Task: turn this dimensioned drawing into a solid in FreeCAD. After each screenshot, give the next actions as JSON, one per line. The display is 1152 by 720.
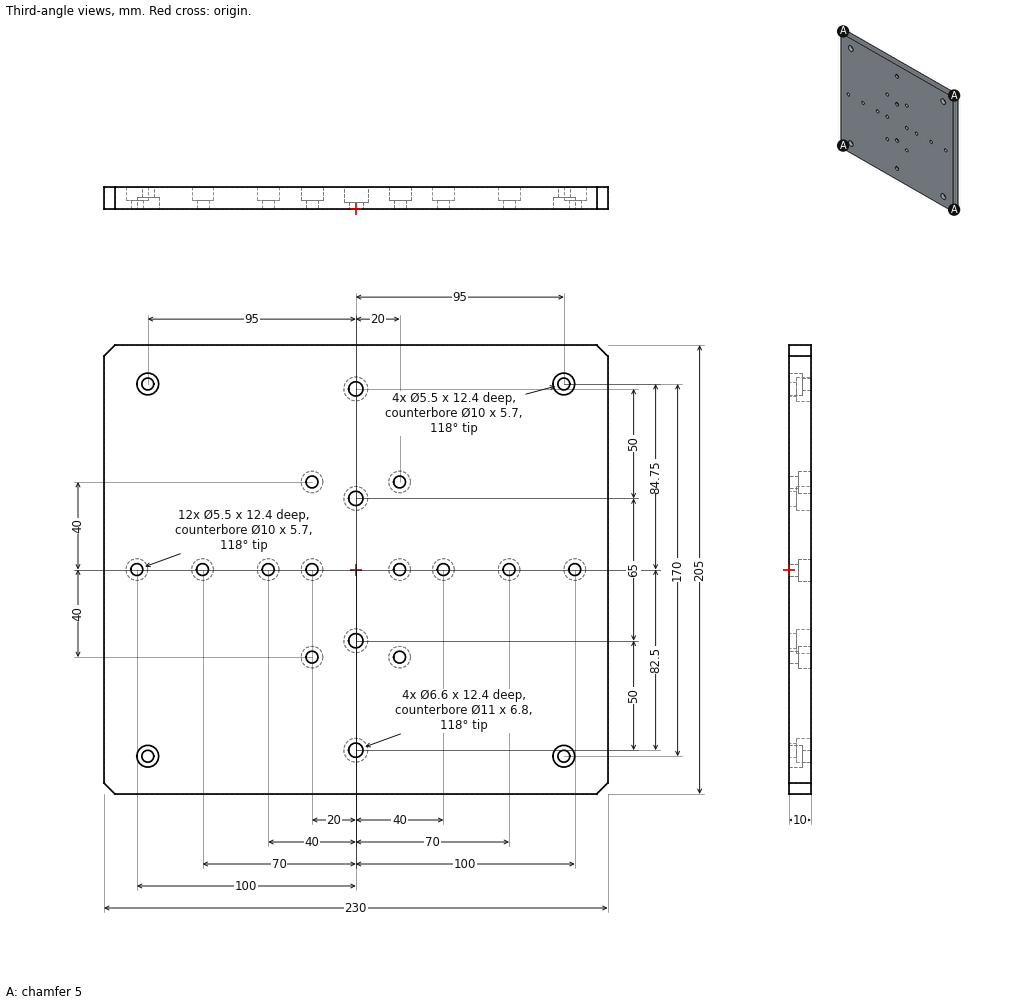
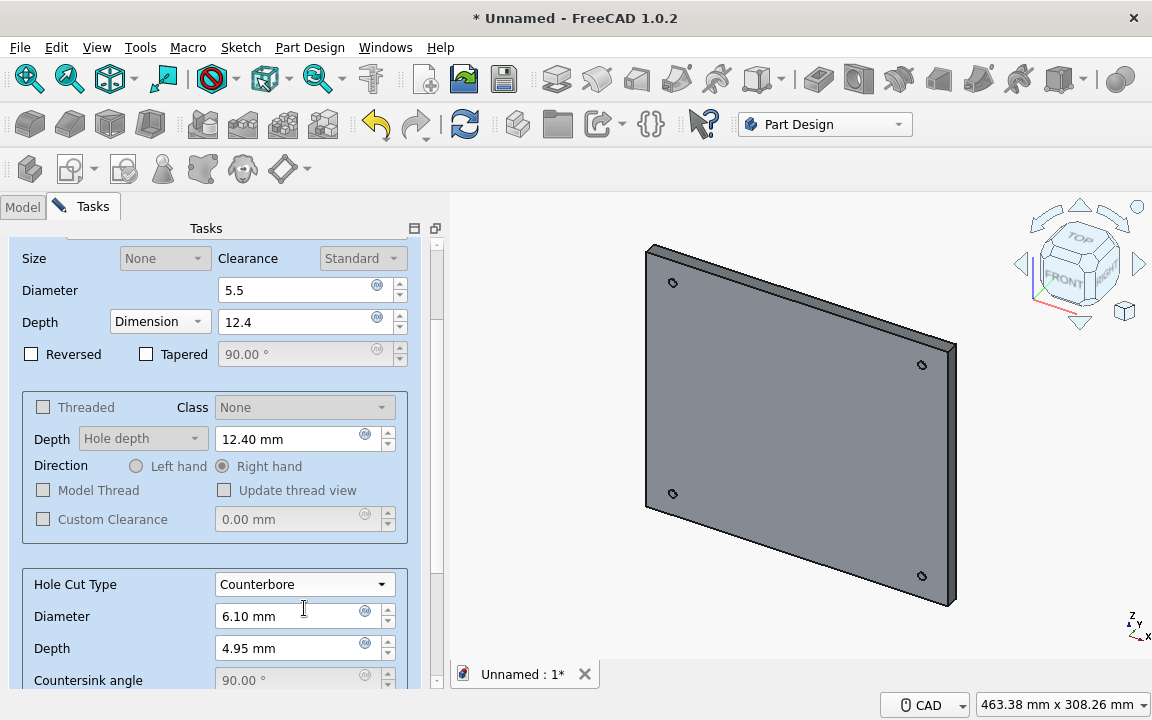
{"action": "triple_click", "coordinate": [298, 616]}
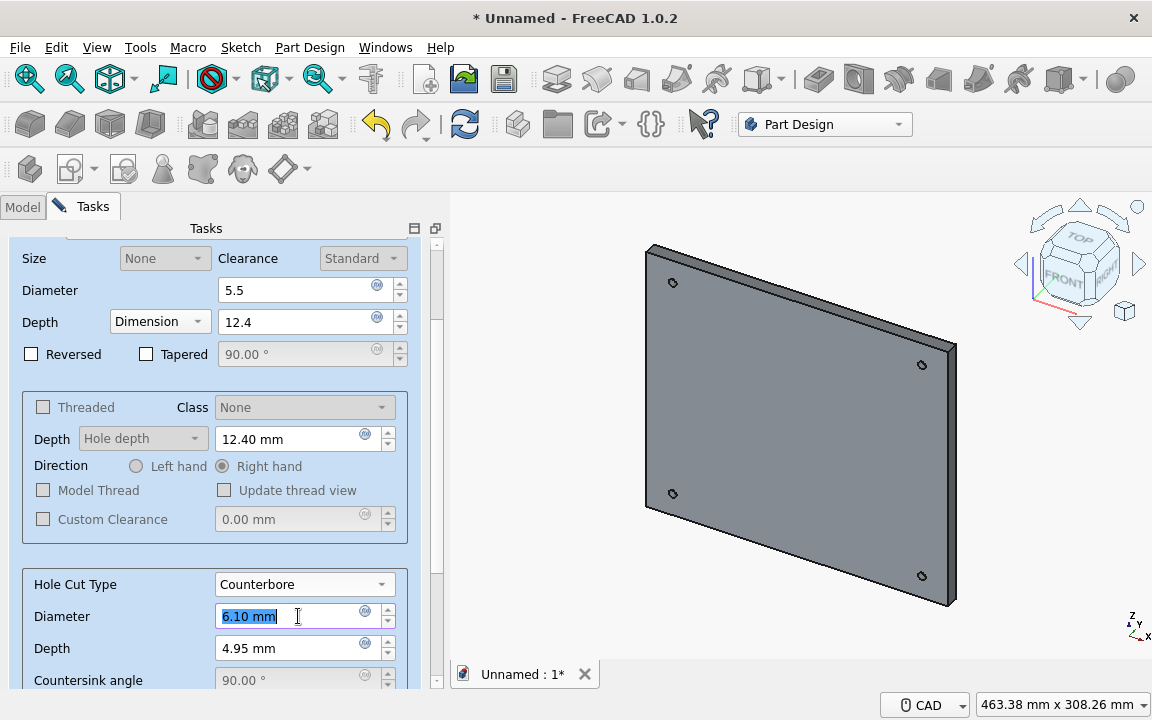
{"action": "type", "text": "10"}
{"action": "key", "text": "Tab"}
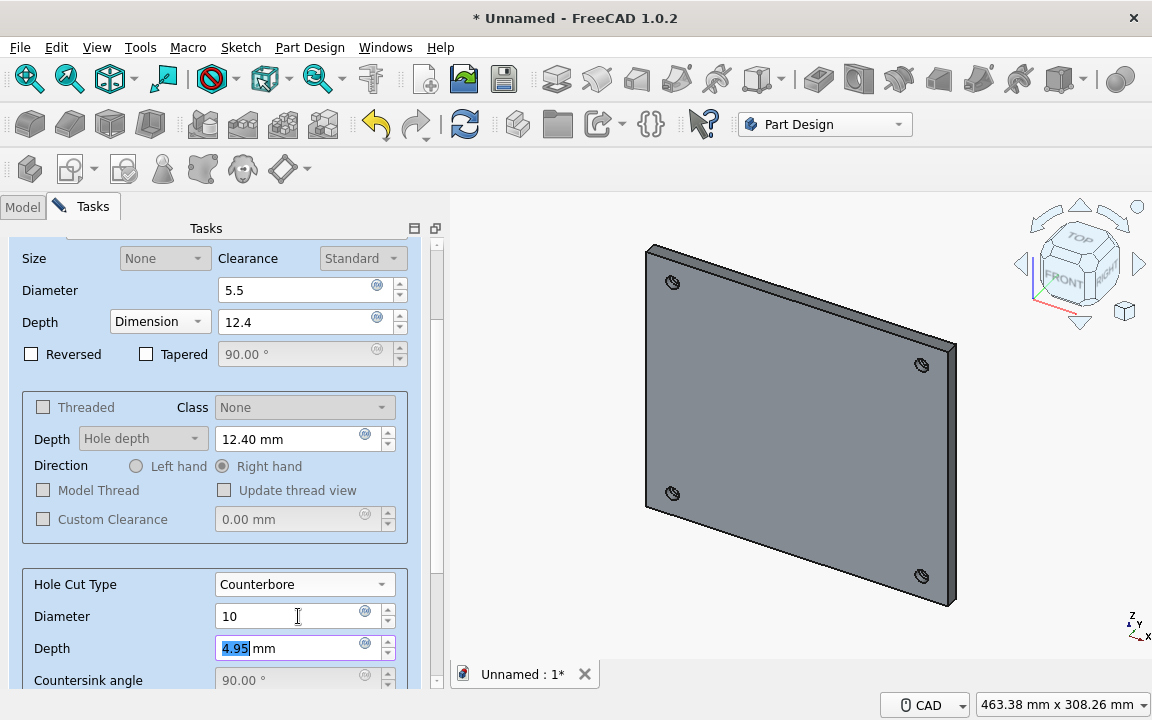
{"action": "type", "text": "5.7"}
{"action": "key", "text": "Tab"}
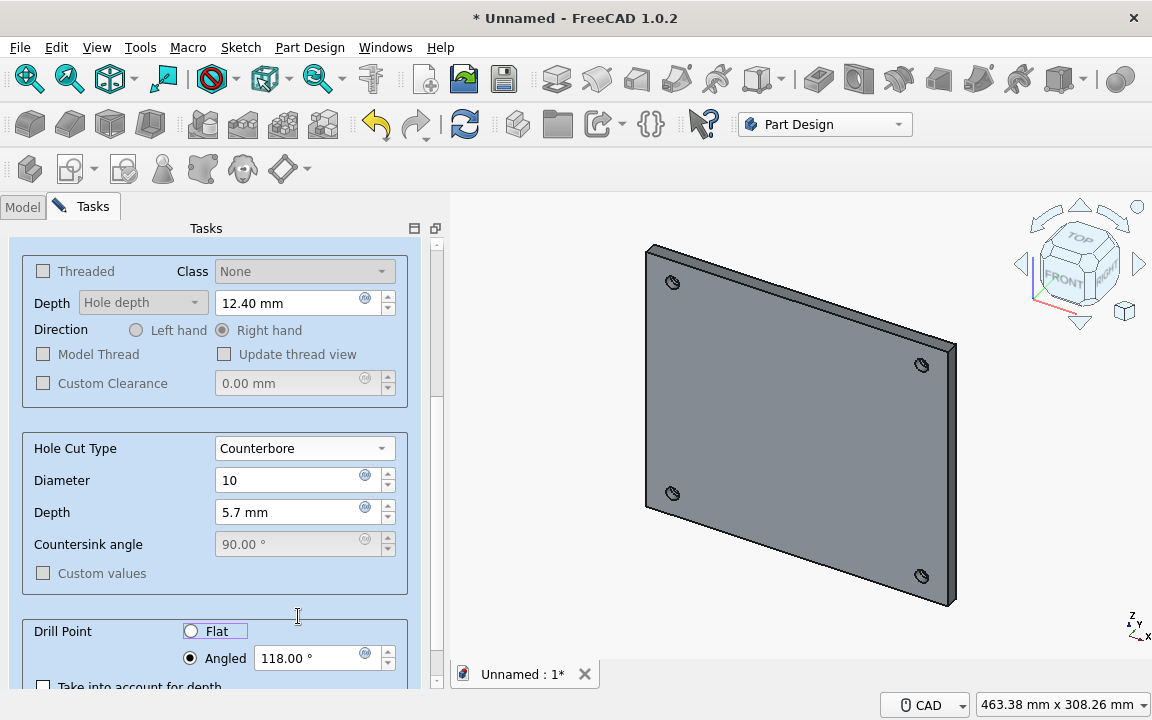
{"action": "scroll", "coordinate": [437, 463], "scroll_direction": "up", "scroll_amount": 6}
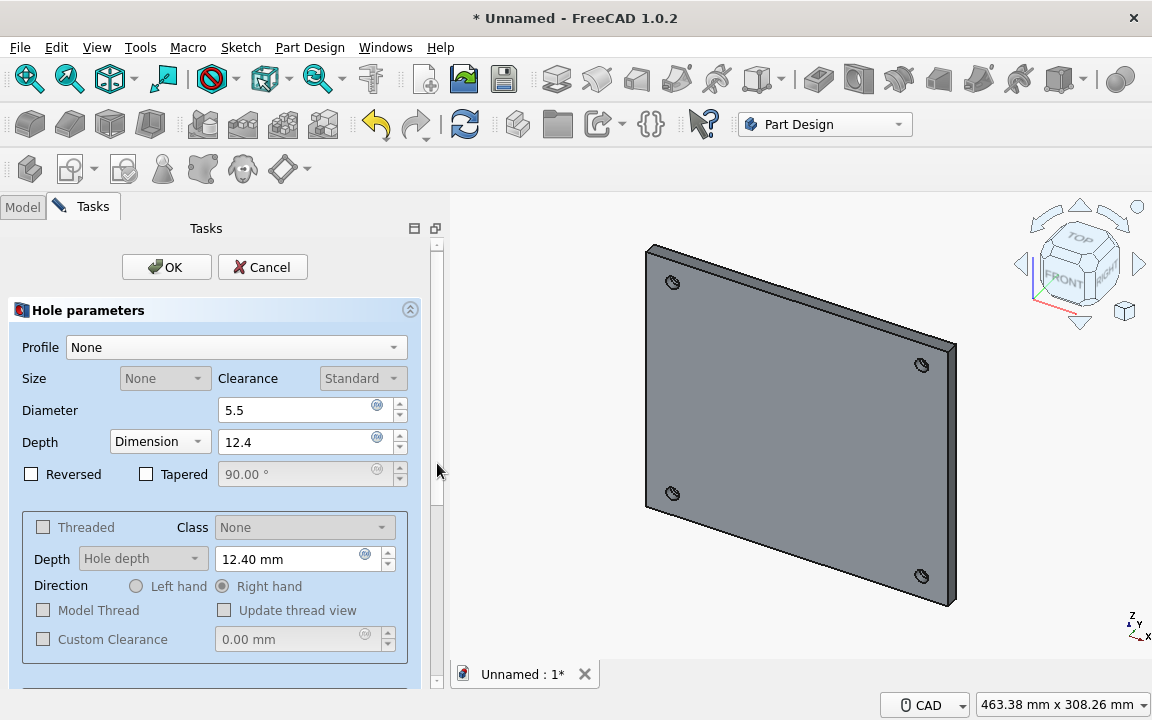
{"action": "left_click", "coordinate": [167, 267]}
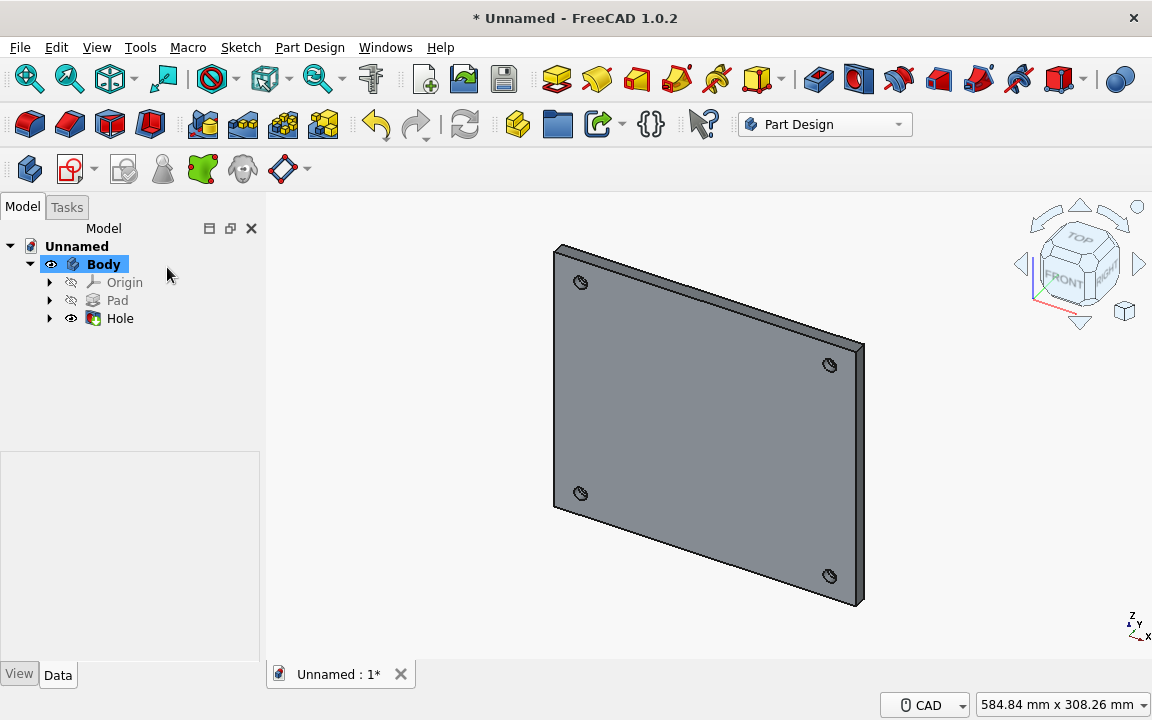
{"action": "key", "text": "4"}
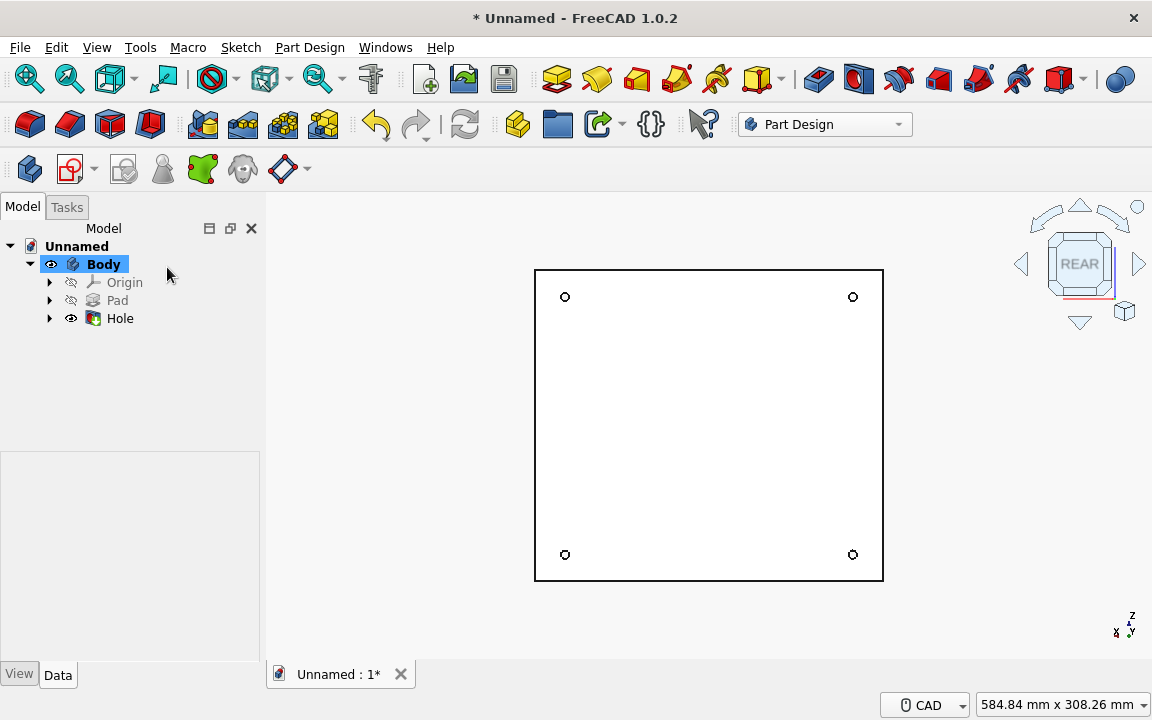
{"action": "left_click", "coordinate": [709, 424]}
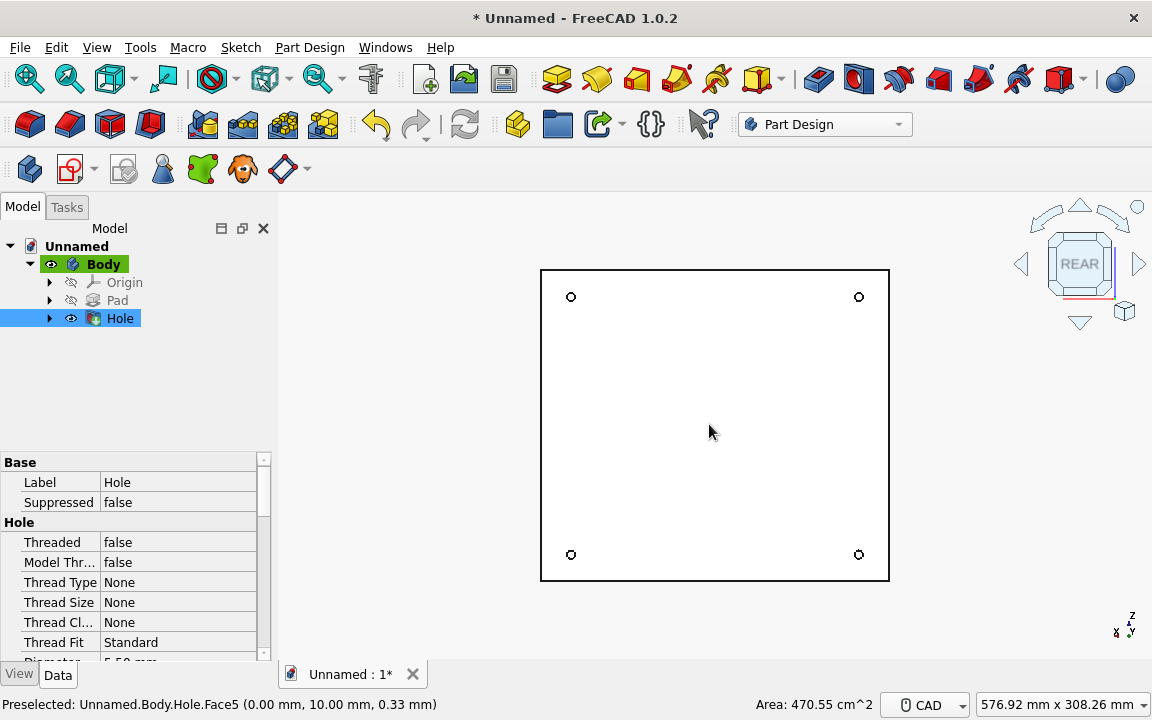
{"action": "left_click", "coordinate": [70, 170]}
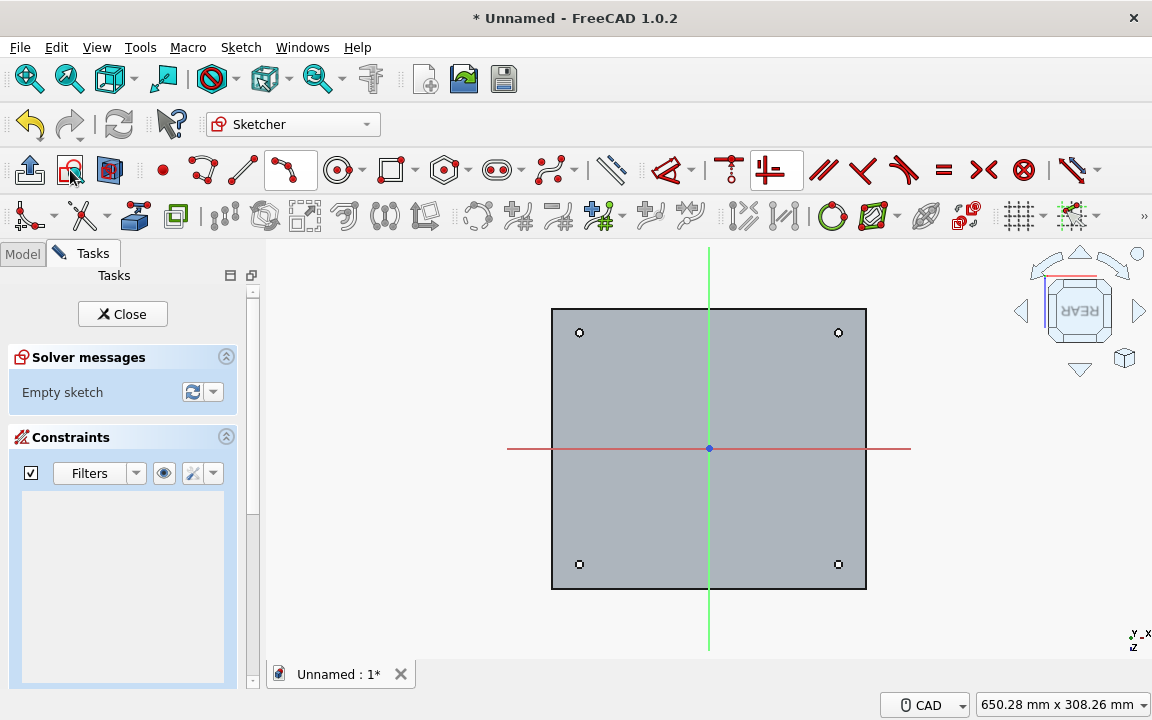
{"action": "scroll", "coordinate": [792, 449], "scroll_direction": "up", "scroll_amount": 3}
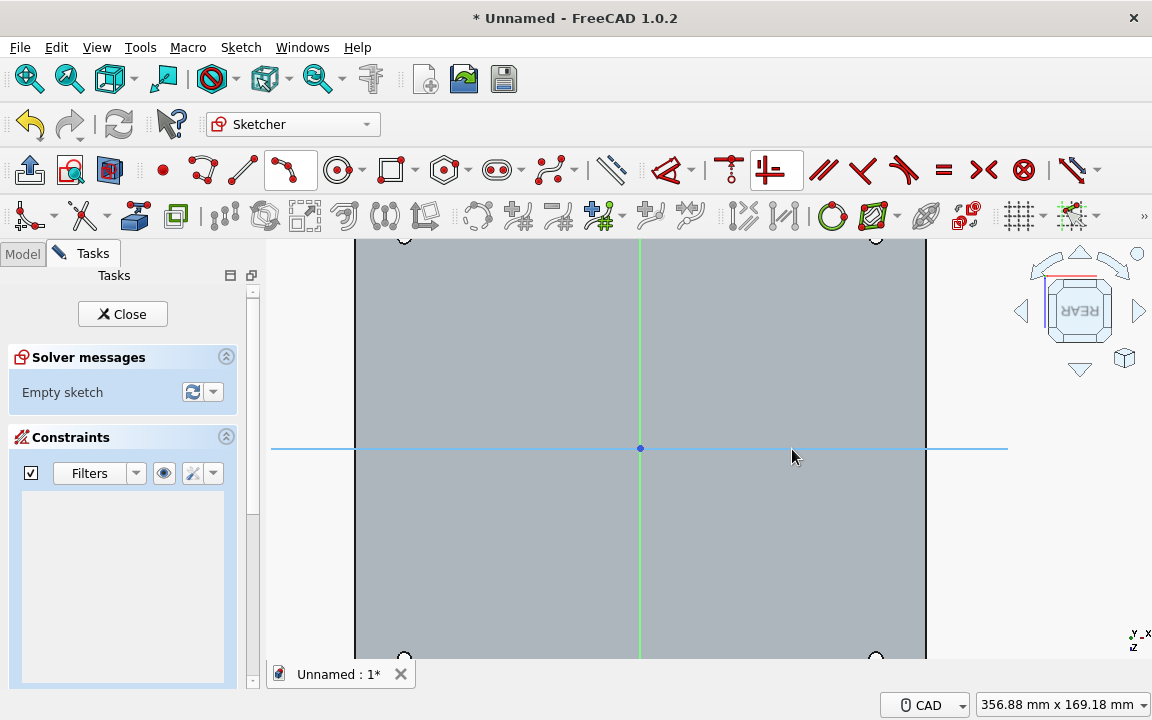
{"action": "left_click", "coordinate": [338, 170]}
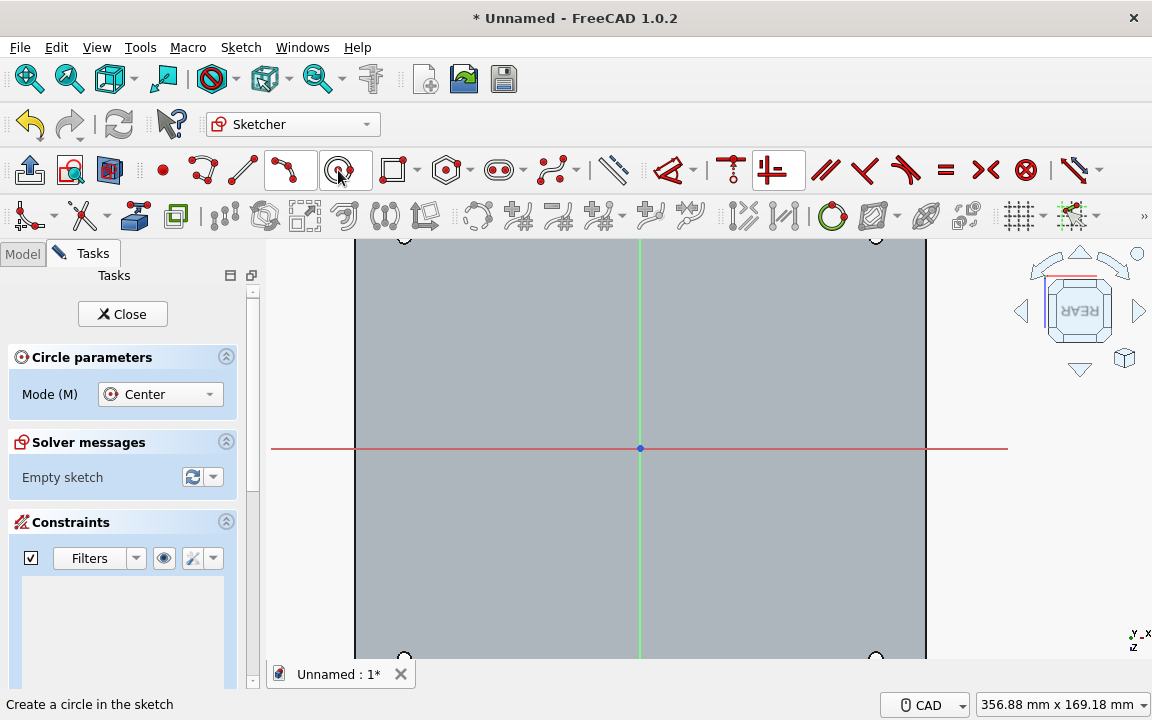
{"action": "scroll", "coordinate": [392, 449], "scroll_direction": "up", "scroll_amount": 7}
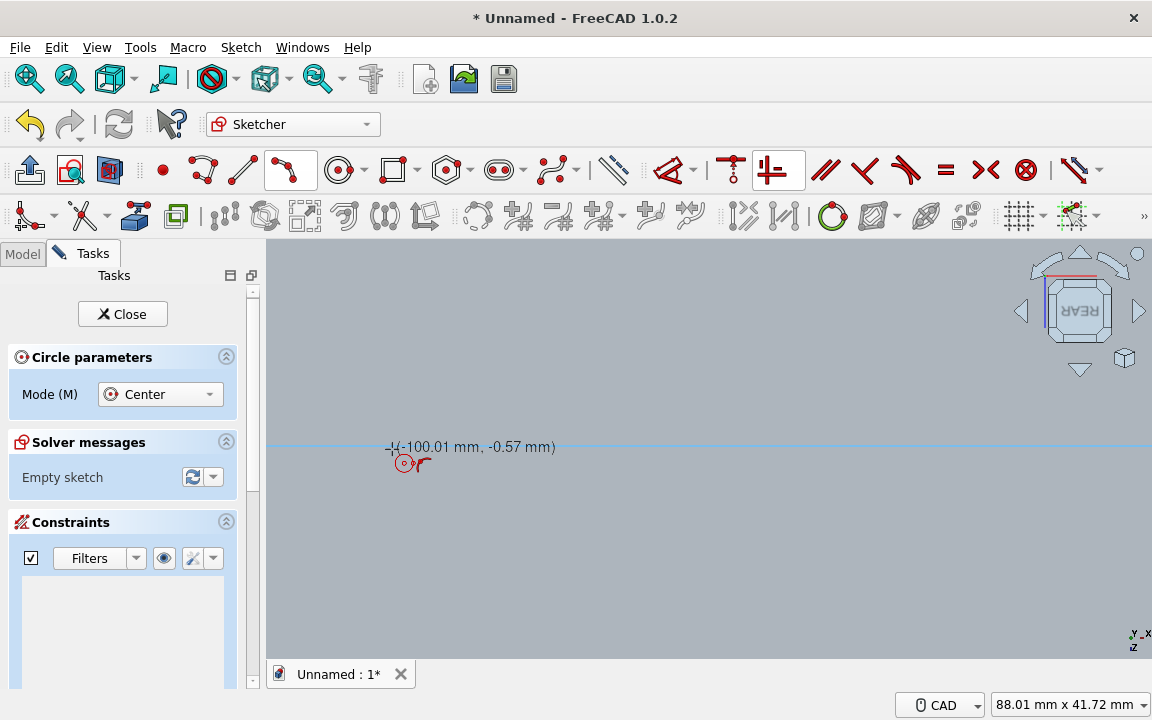
{"action": "scroll", "coordinate": [392, 450], "scroll_direction": "down", "scroll_amount": 7}